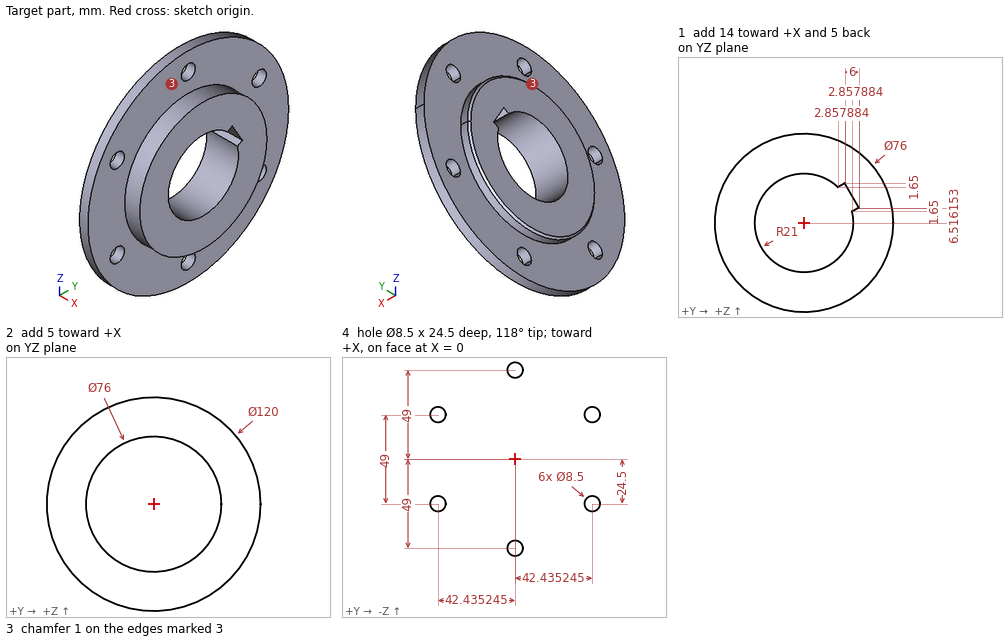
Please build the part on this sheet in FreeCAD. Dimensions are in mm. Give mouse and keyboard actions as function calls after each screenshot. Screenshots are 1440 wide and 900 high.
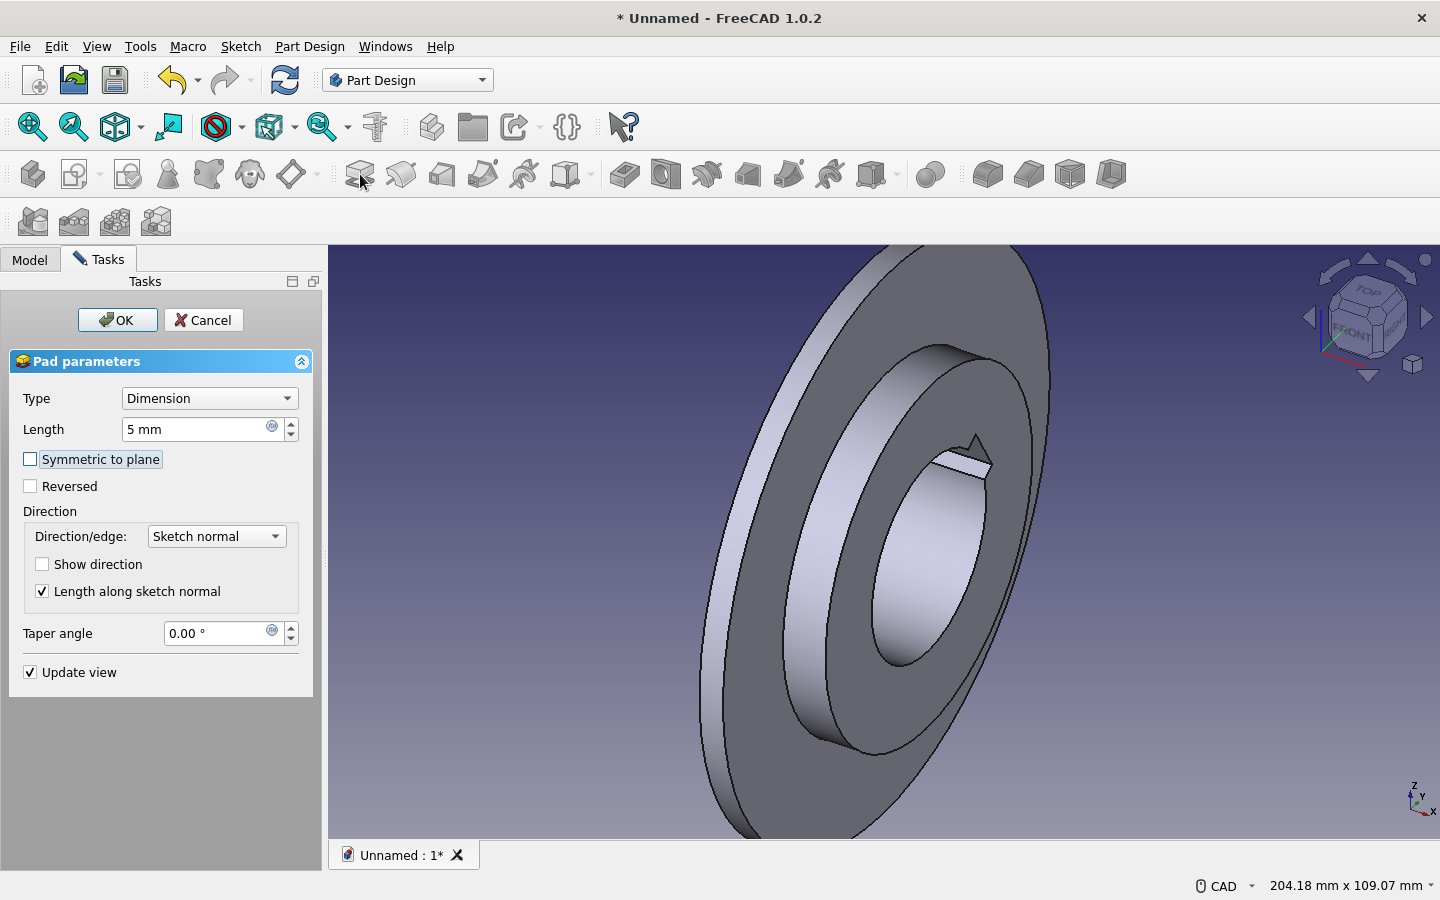
click(118, 320)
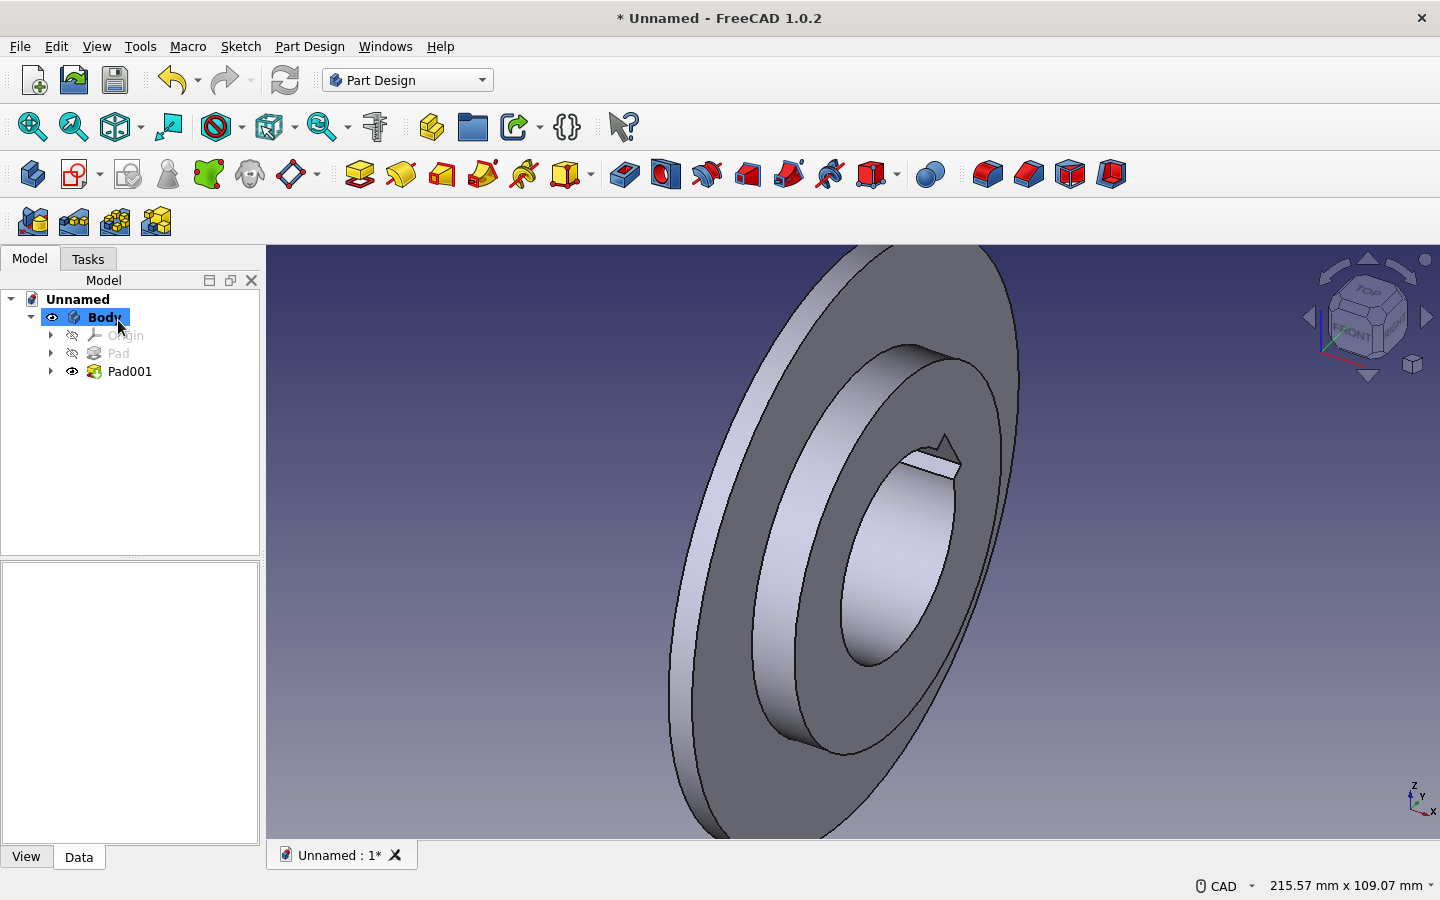
click(33, 128)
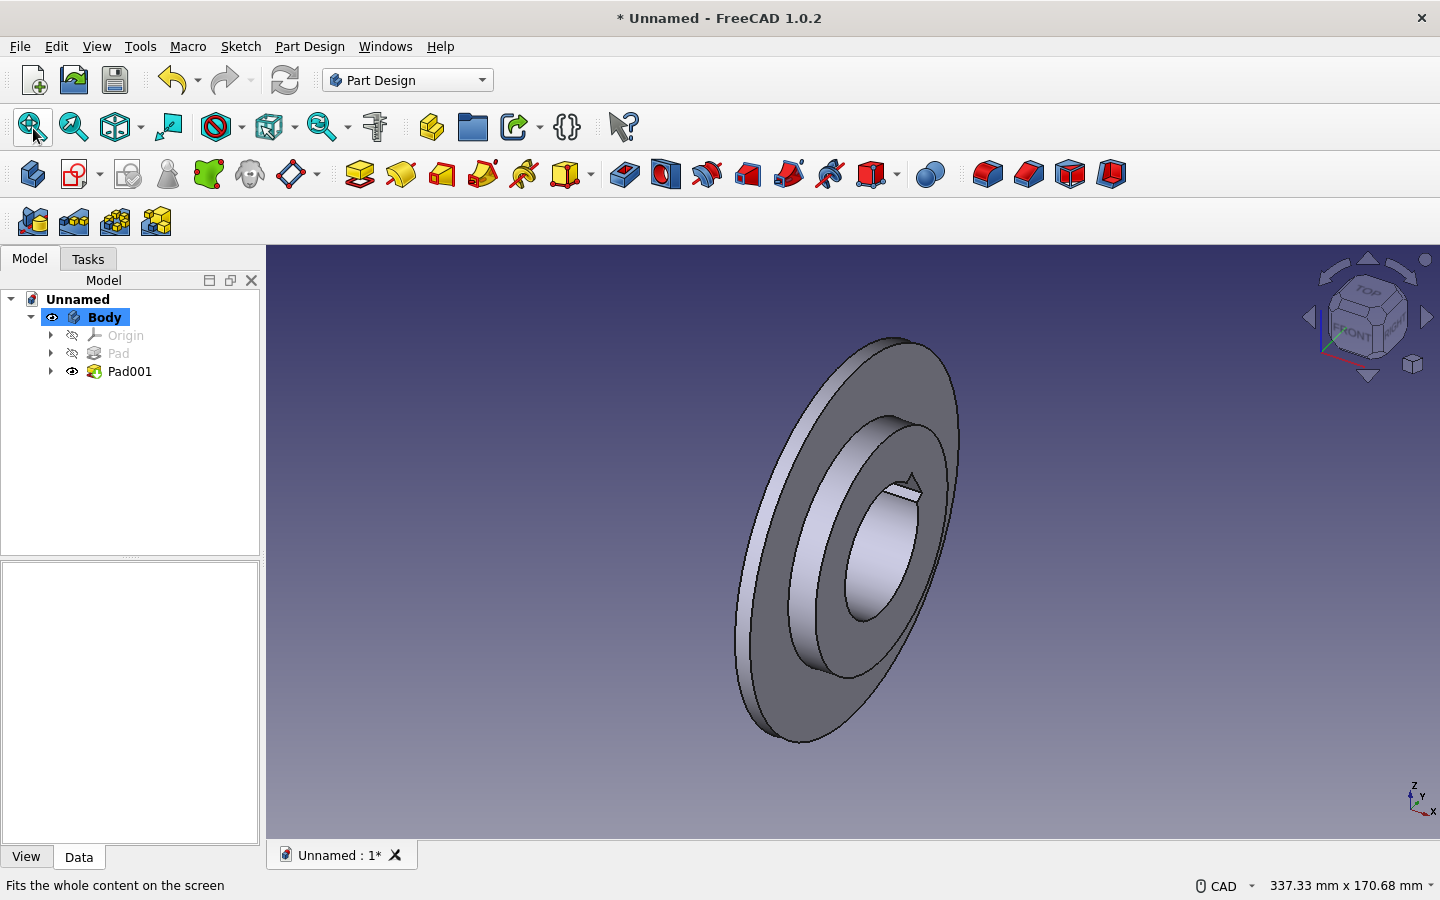
key(0)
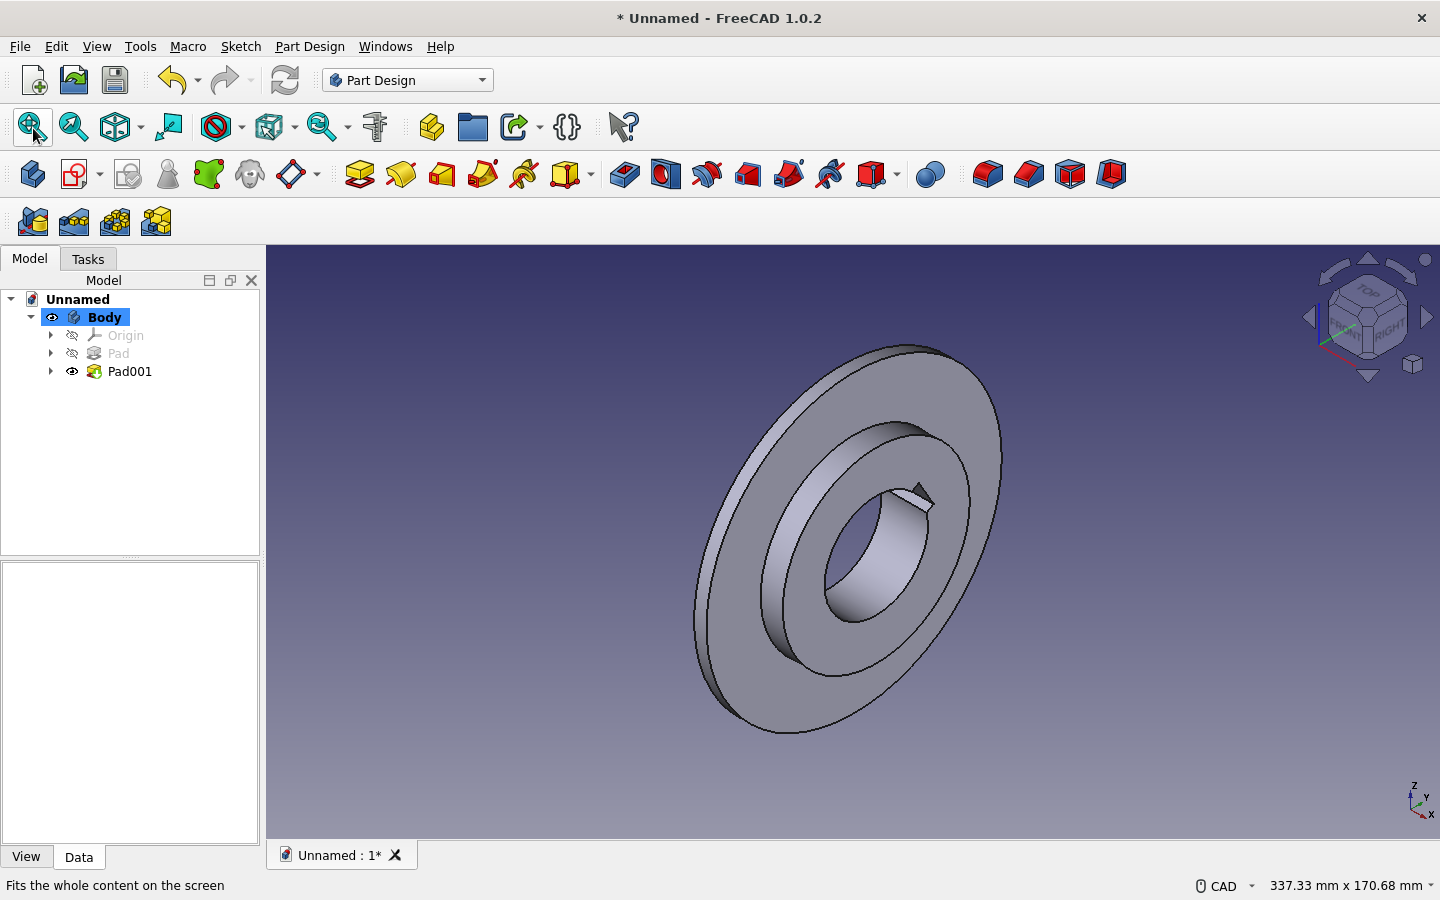
key(2)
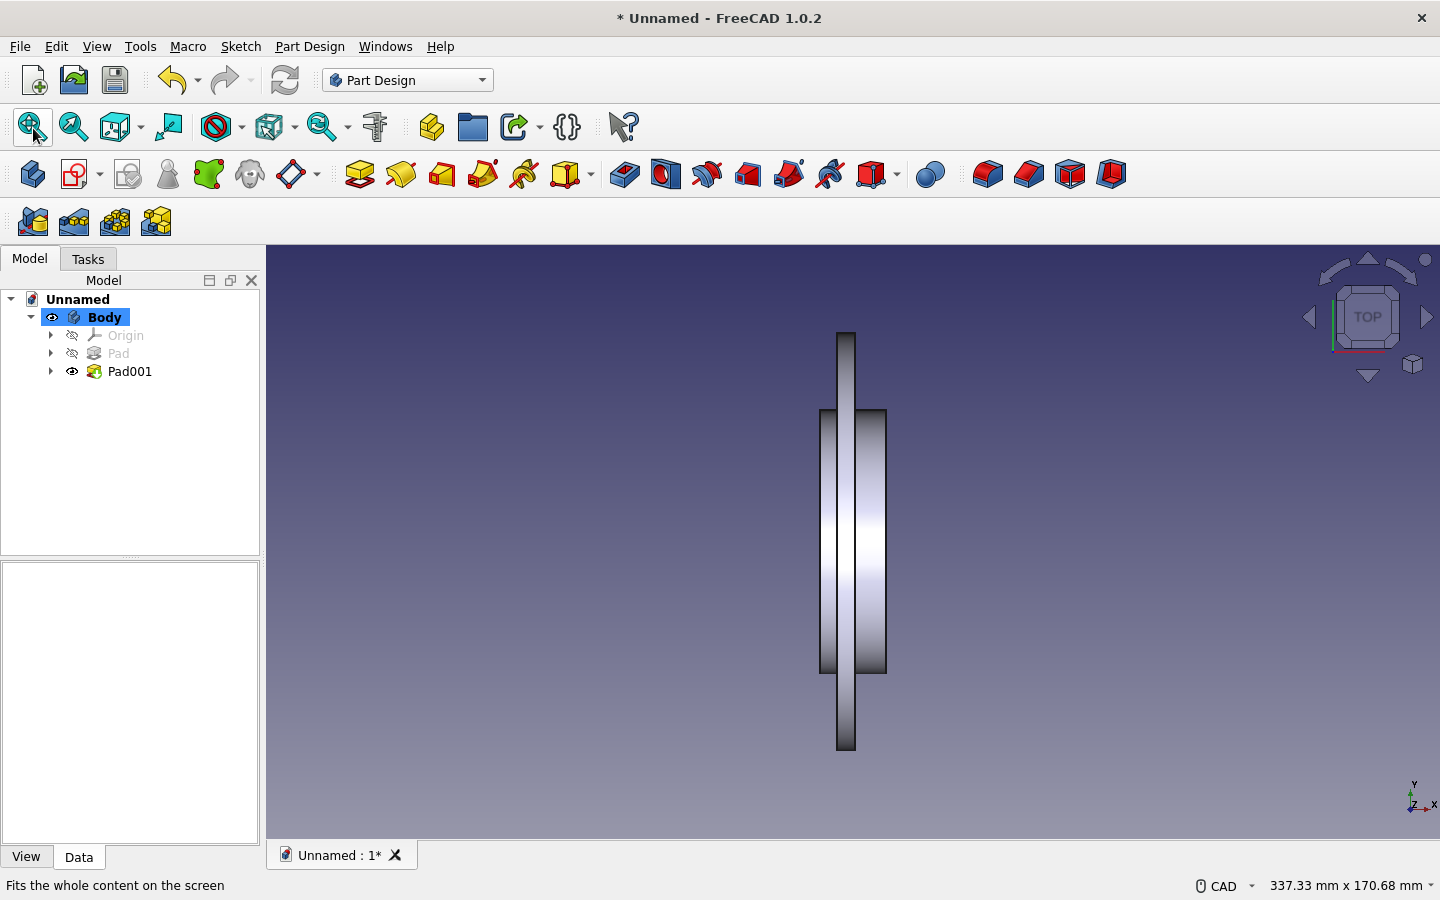
click(820, 648)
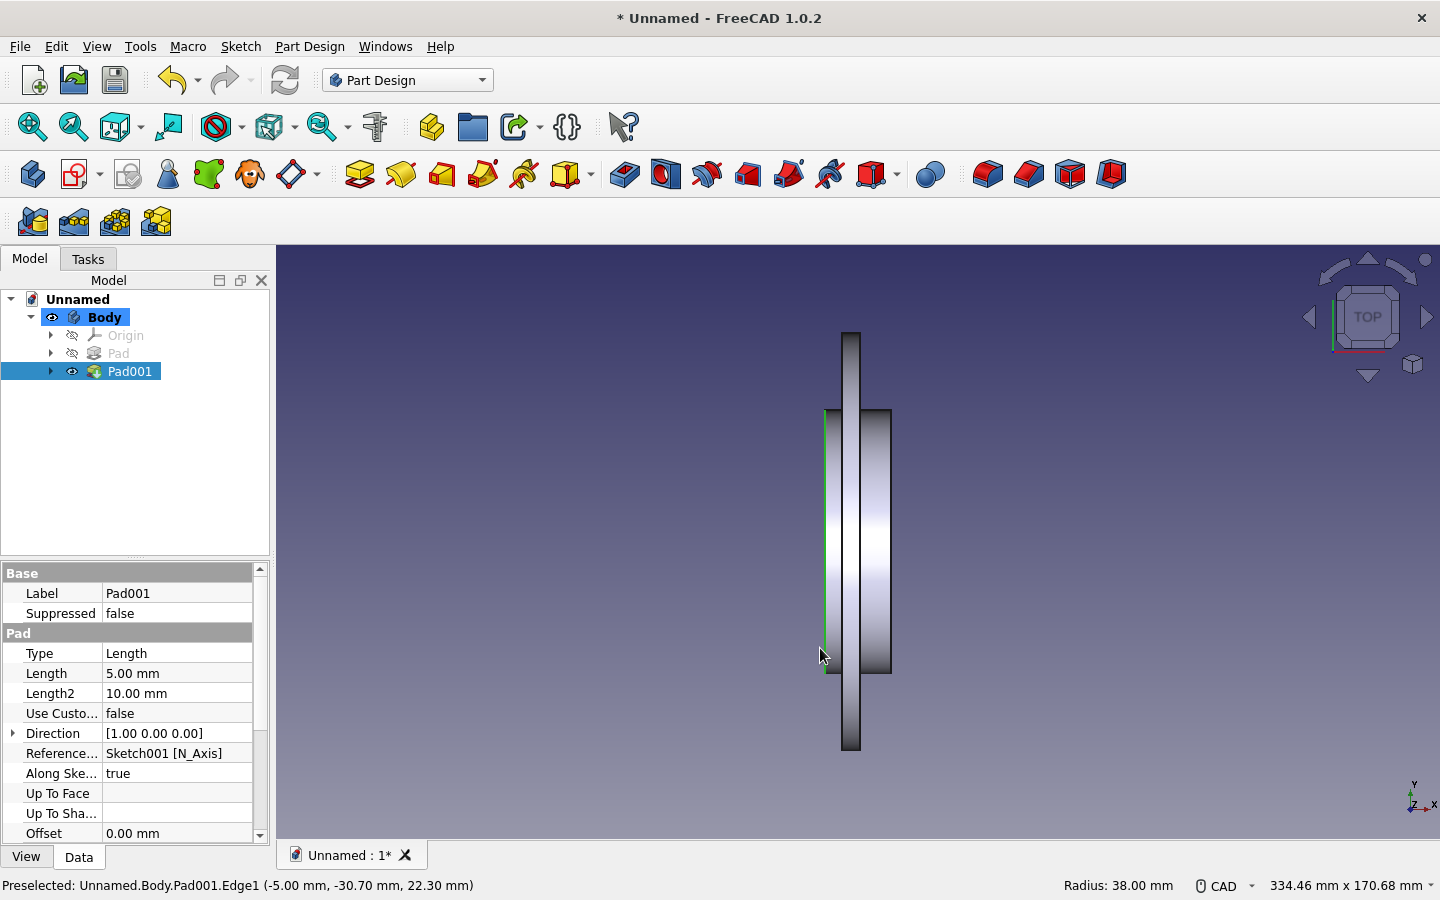
click(1029, 174)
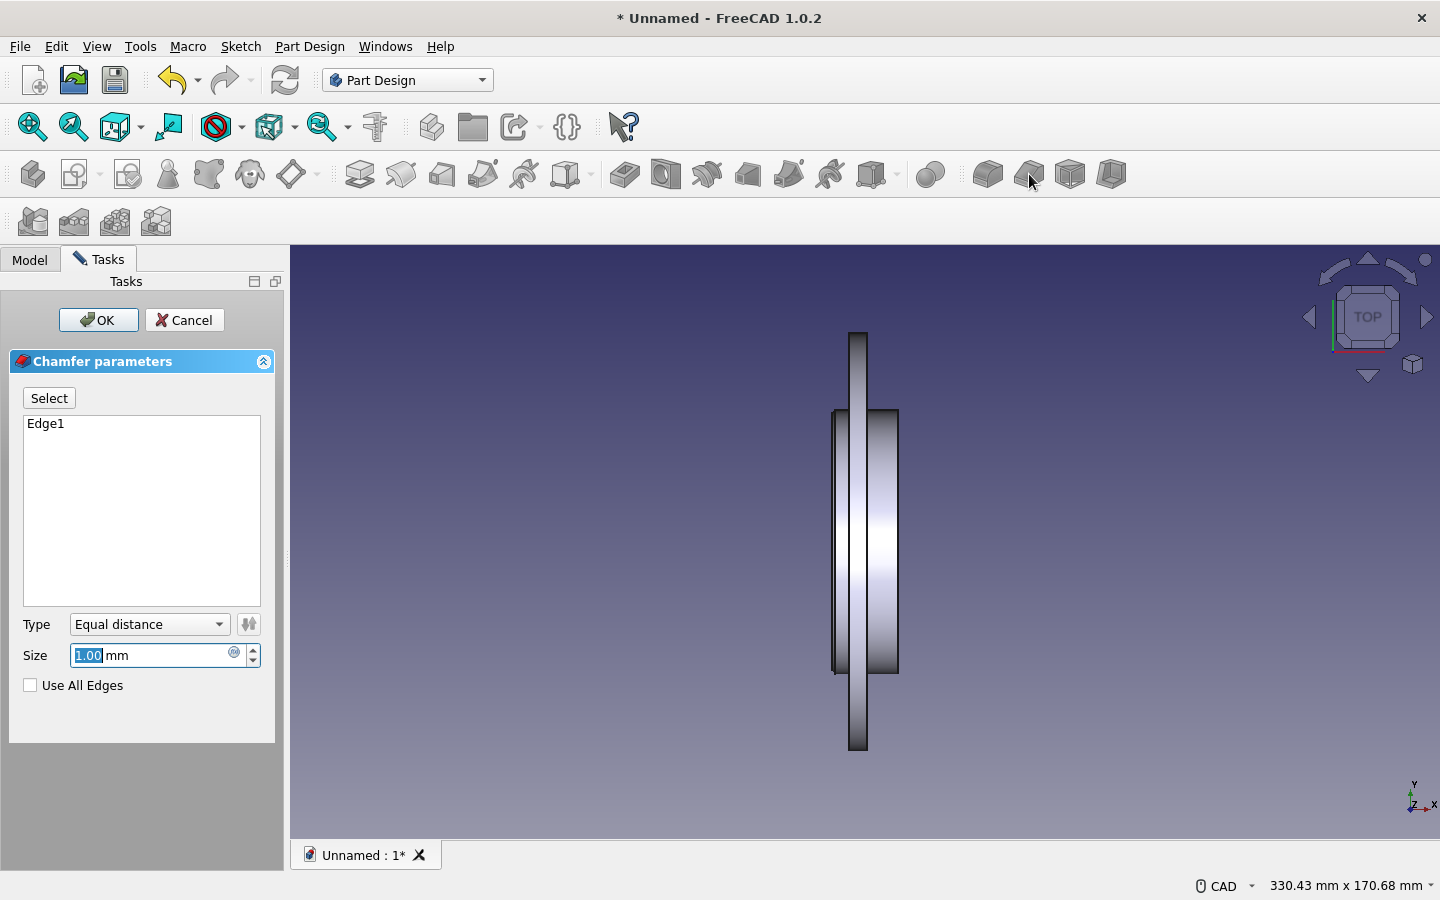
text(1)
key(Tab)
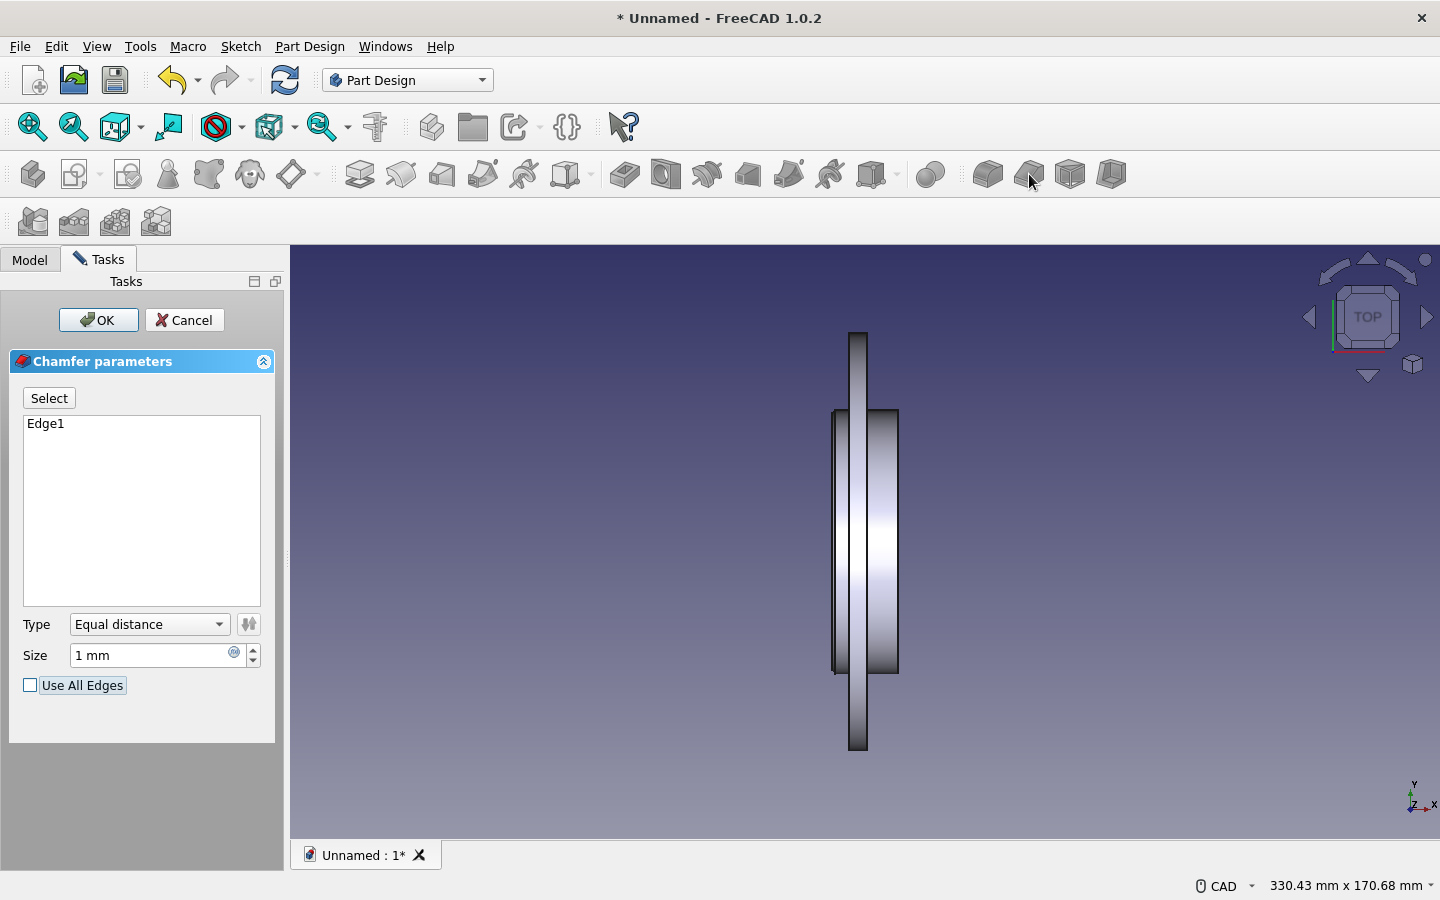
click(99, 320)